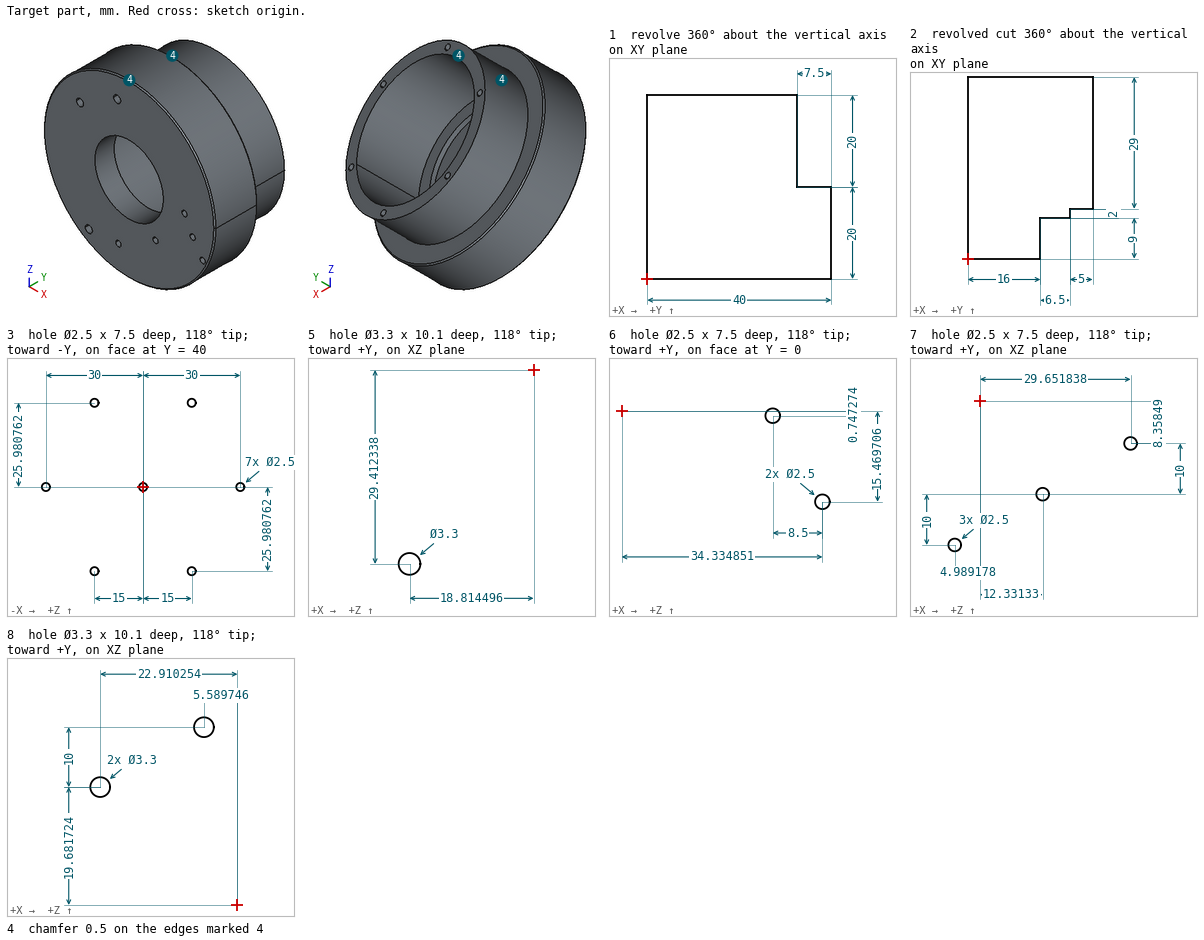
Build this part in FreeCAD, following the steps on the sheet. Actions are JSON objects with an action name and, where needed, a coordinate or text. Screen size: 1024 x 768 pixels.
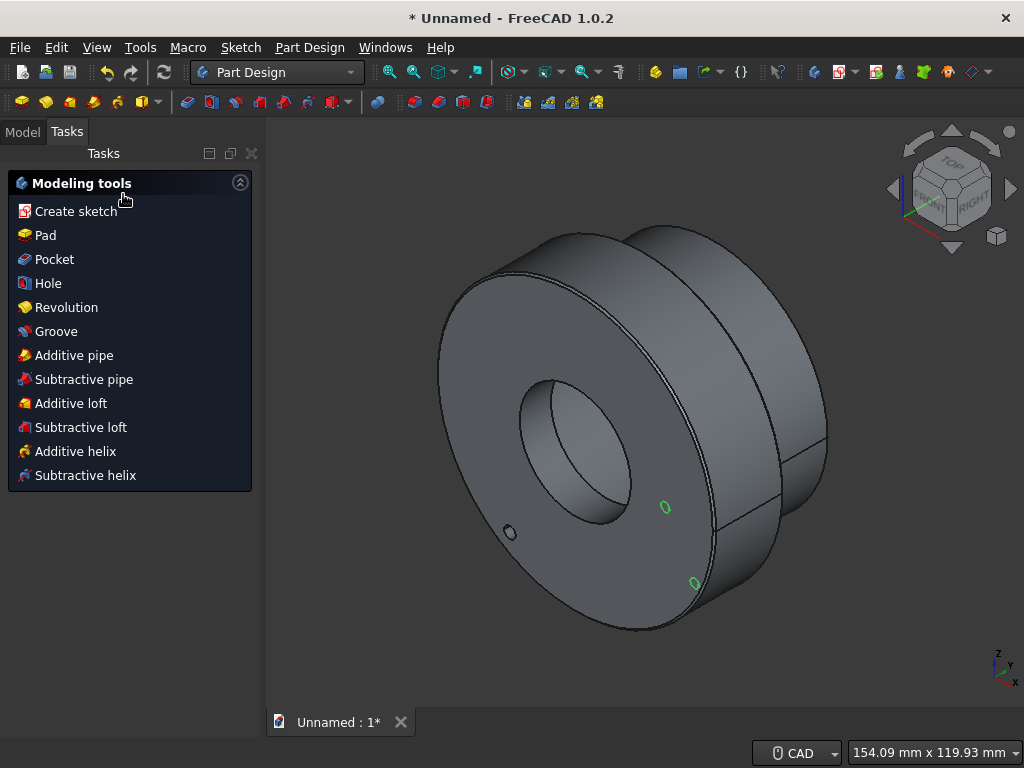
{"action": "left_click", "coordinate": [212, 102]}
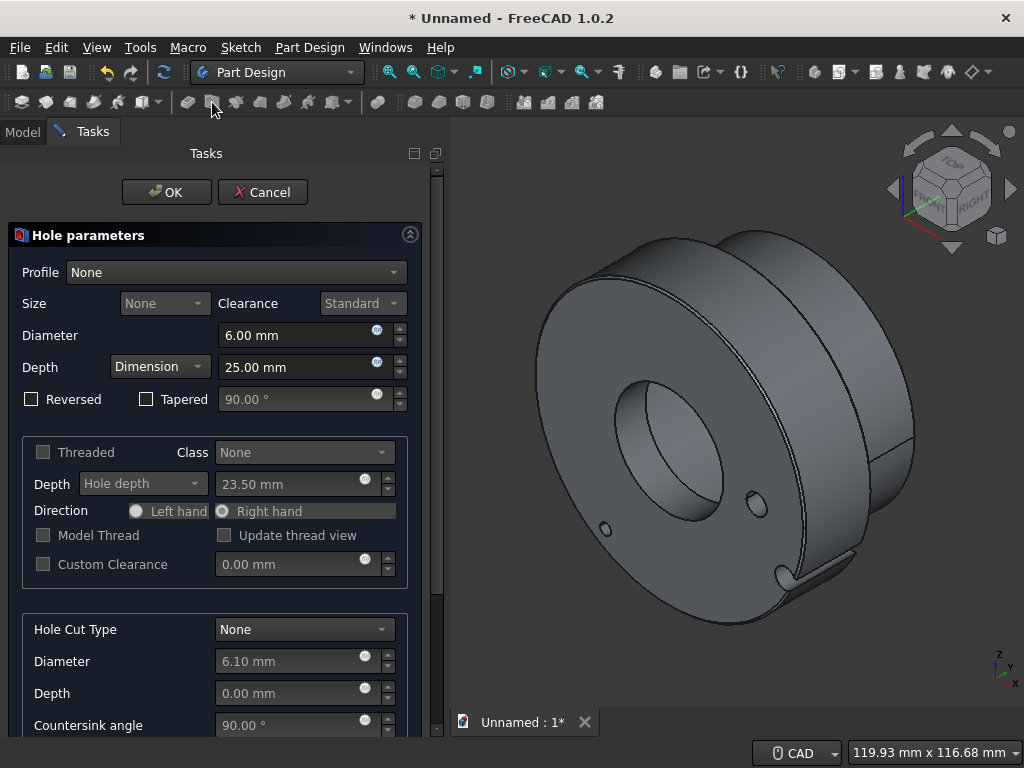
{"action": "triple_click", "coordinate": [305, 335]}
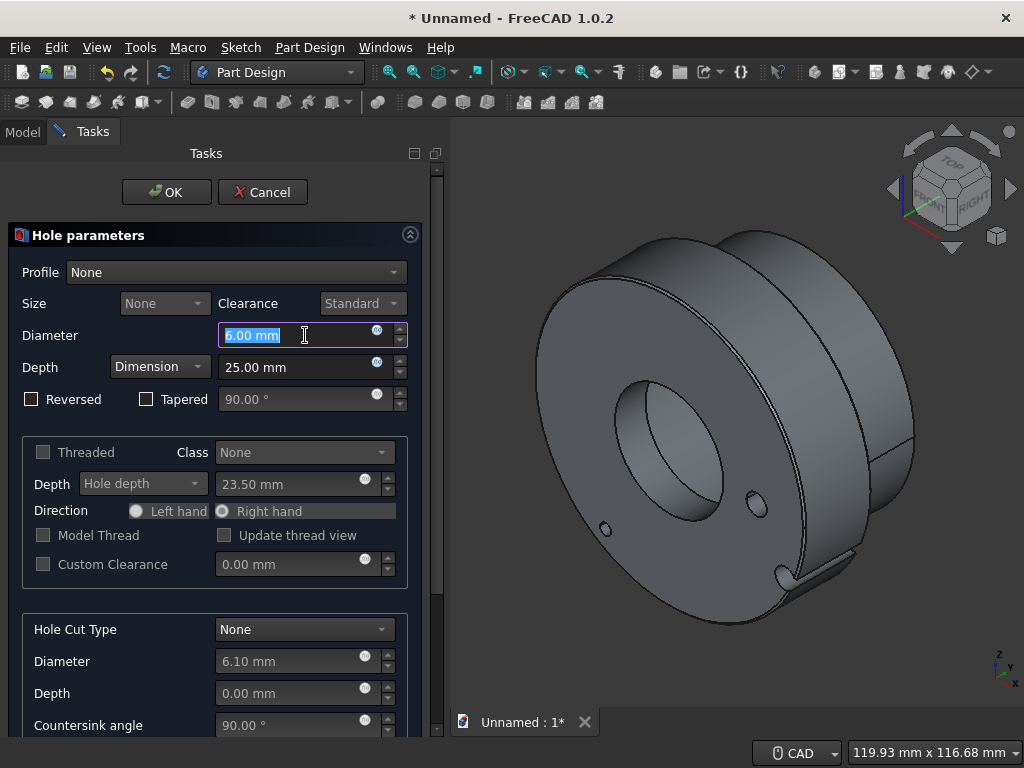
{"action": "type", "text": "2.5"}
{"action": "key", "text": "Tab"}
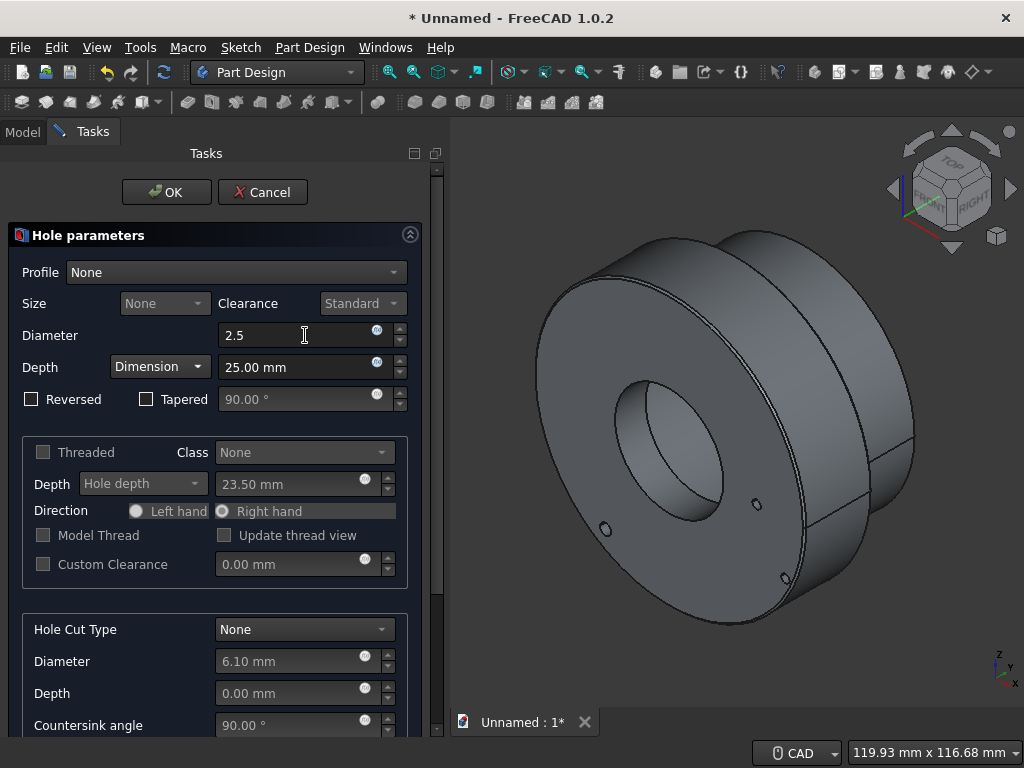
{"action": "triple_click", "coordinate": [305, 367]}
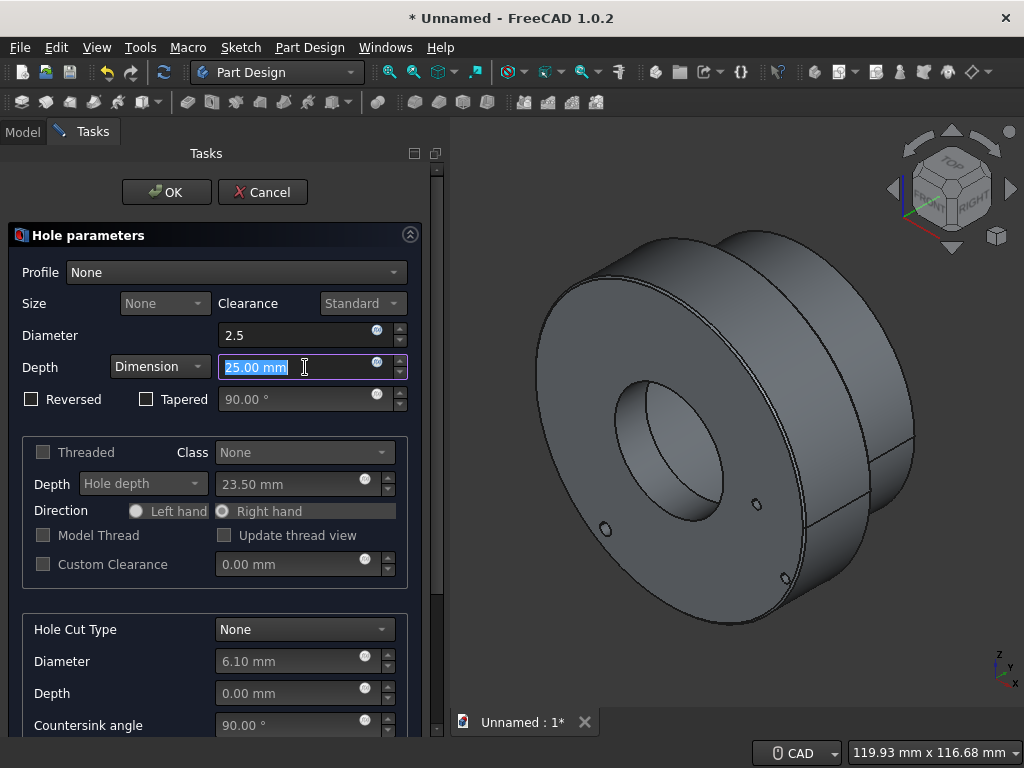
{"action": "type", "text": "7.5"}
{"action": "key", "text": "Tab"}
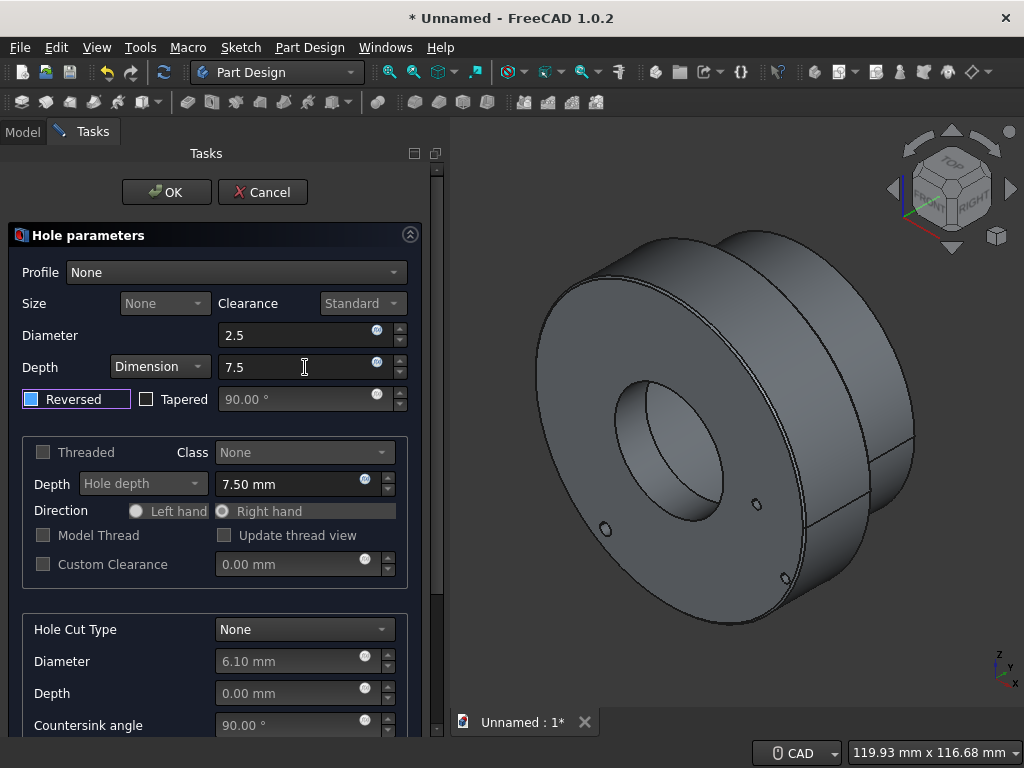
{"action": "left_click", "coordinate": [167, 192]}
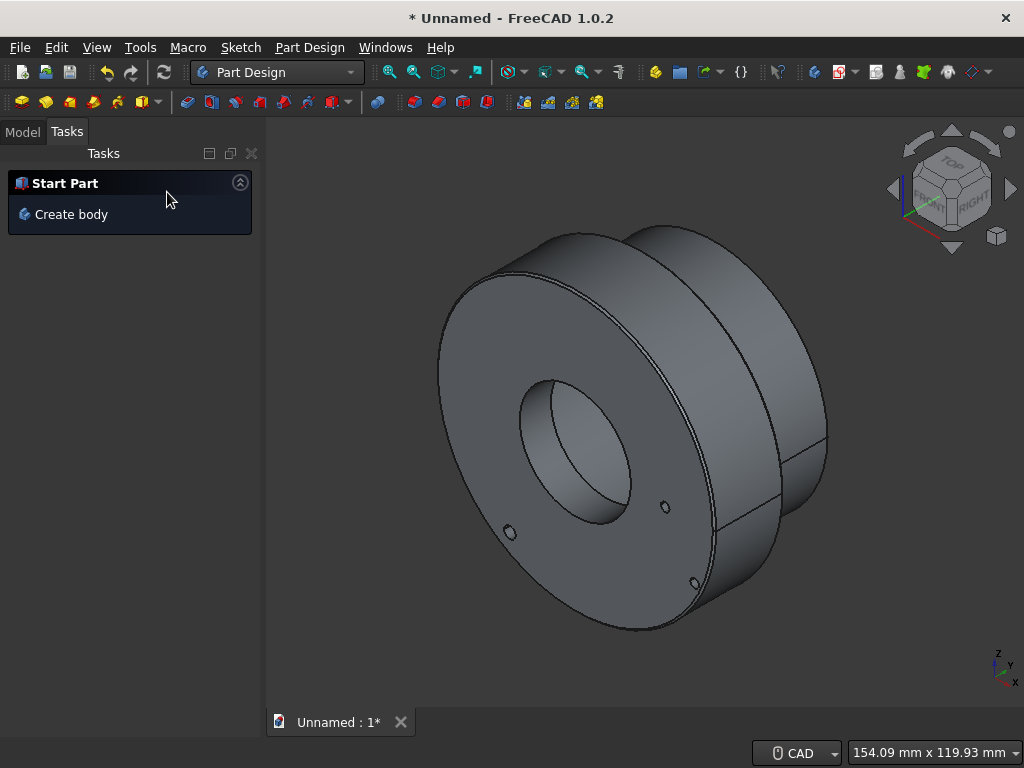
{"action": "left_click", "coordinate": [840, 72]}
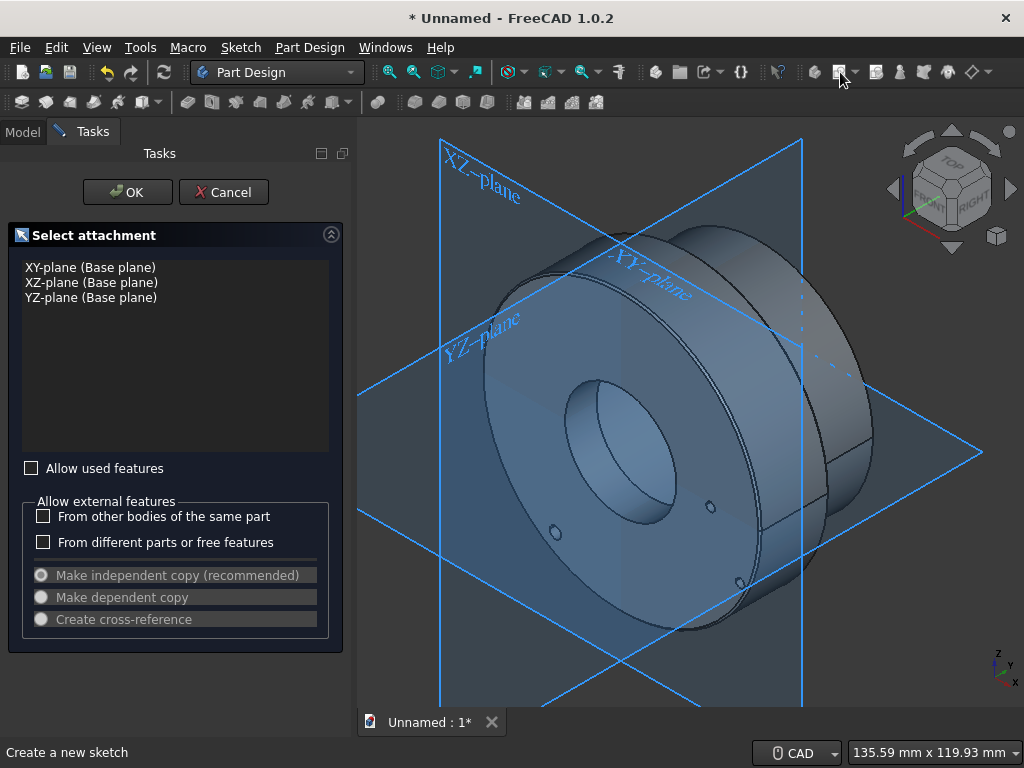
{"action": "left_click", "coordinate": [82, 282]}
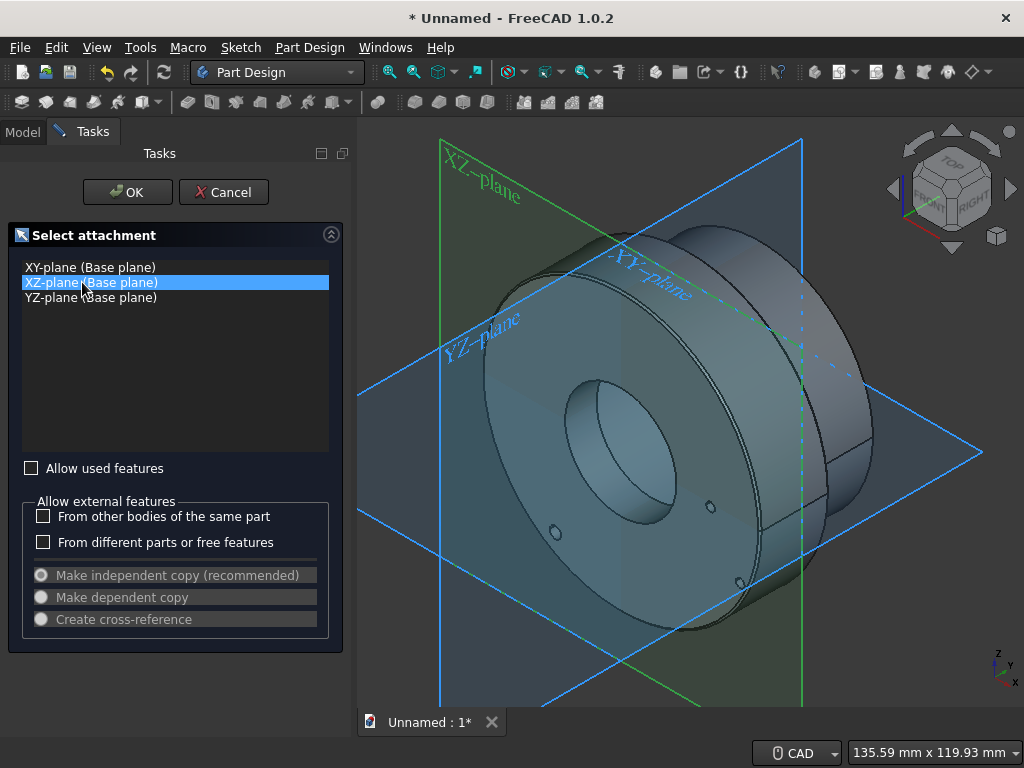
{"action": "left_click", "coordinate": [128, 192]}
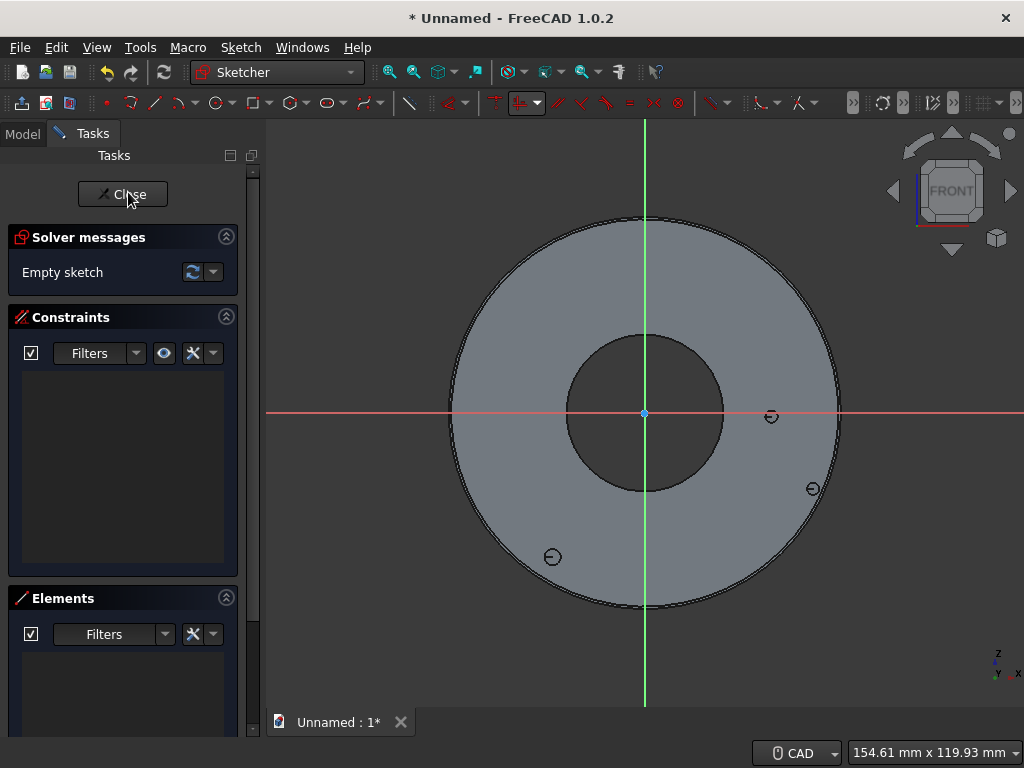
{"action": "scroll", "coordinate": [810, 545], "scroll_direction": "up", "scroll_amount": 4}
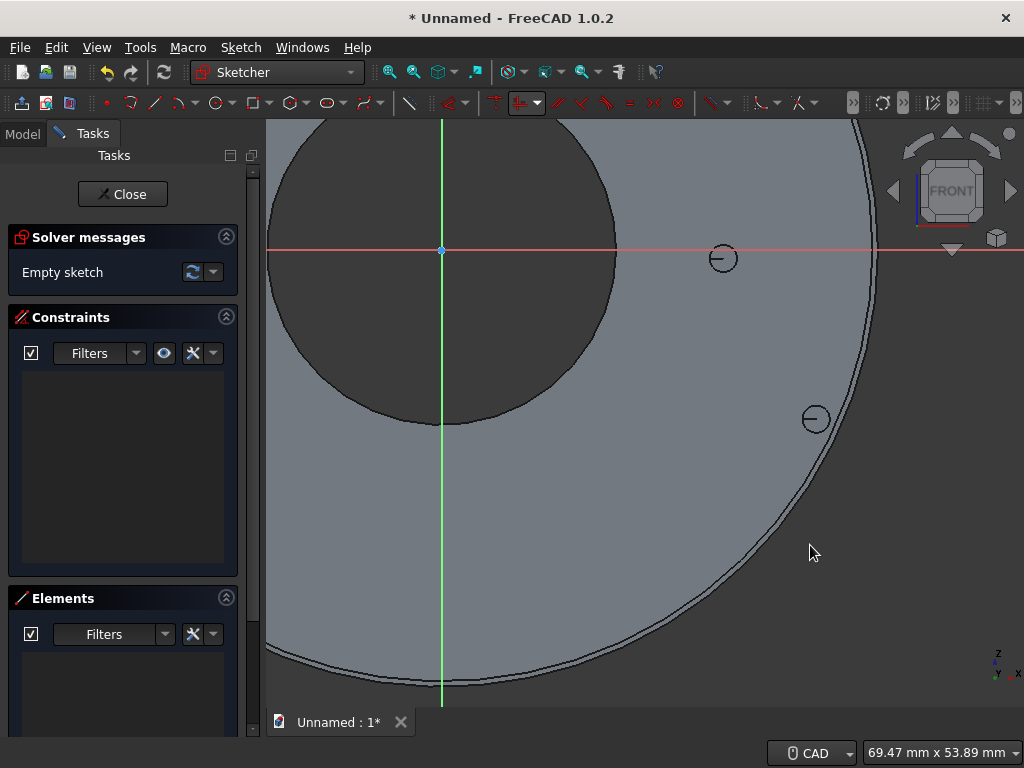
{"action": "left_click", "coordinate": [216, 104]}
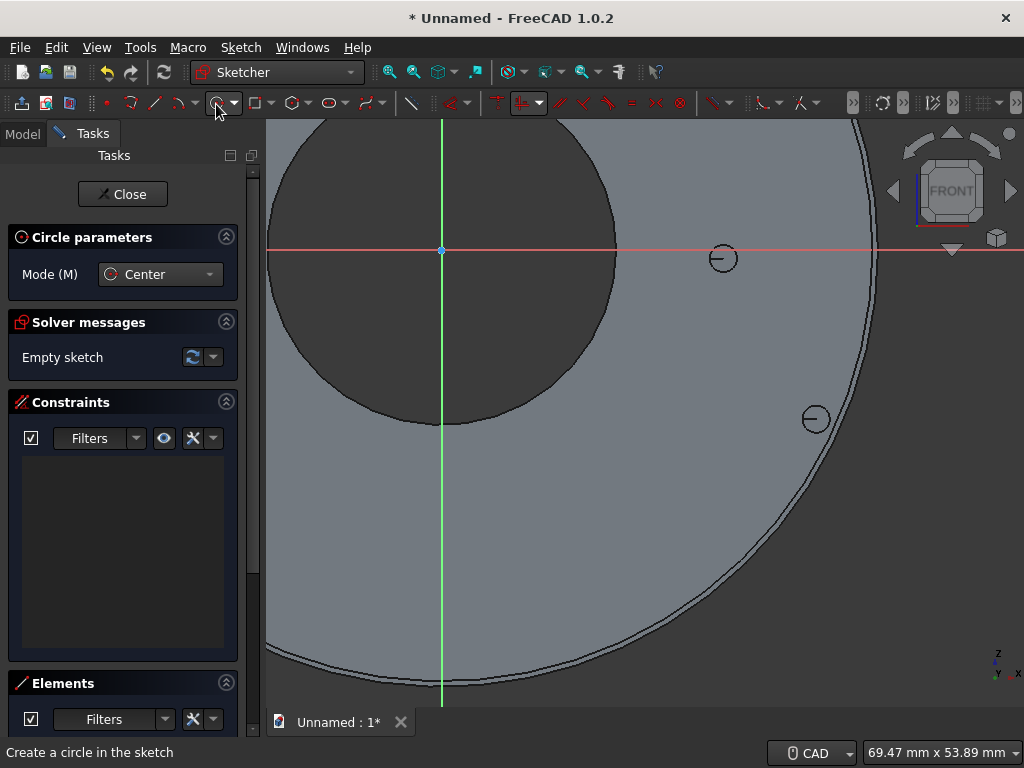
{"action": "scroll", "coordinate": [387, 560], "scroll_direction": "up", "scroll_amount": 3}